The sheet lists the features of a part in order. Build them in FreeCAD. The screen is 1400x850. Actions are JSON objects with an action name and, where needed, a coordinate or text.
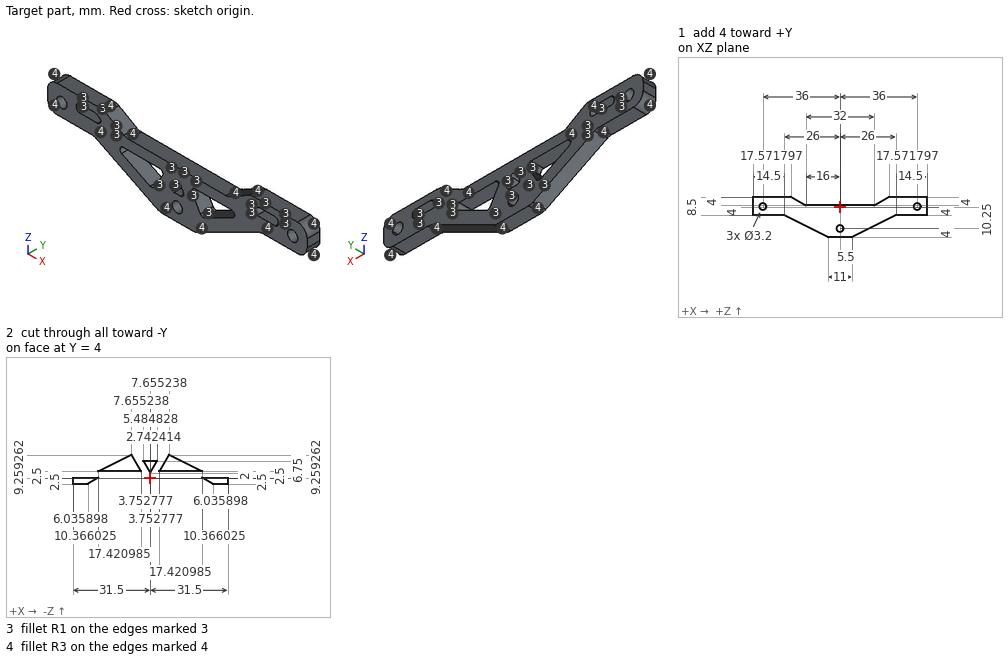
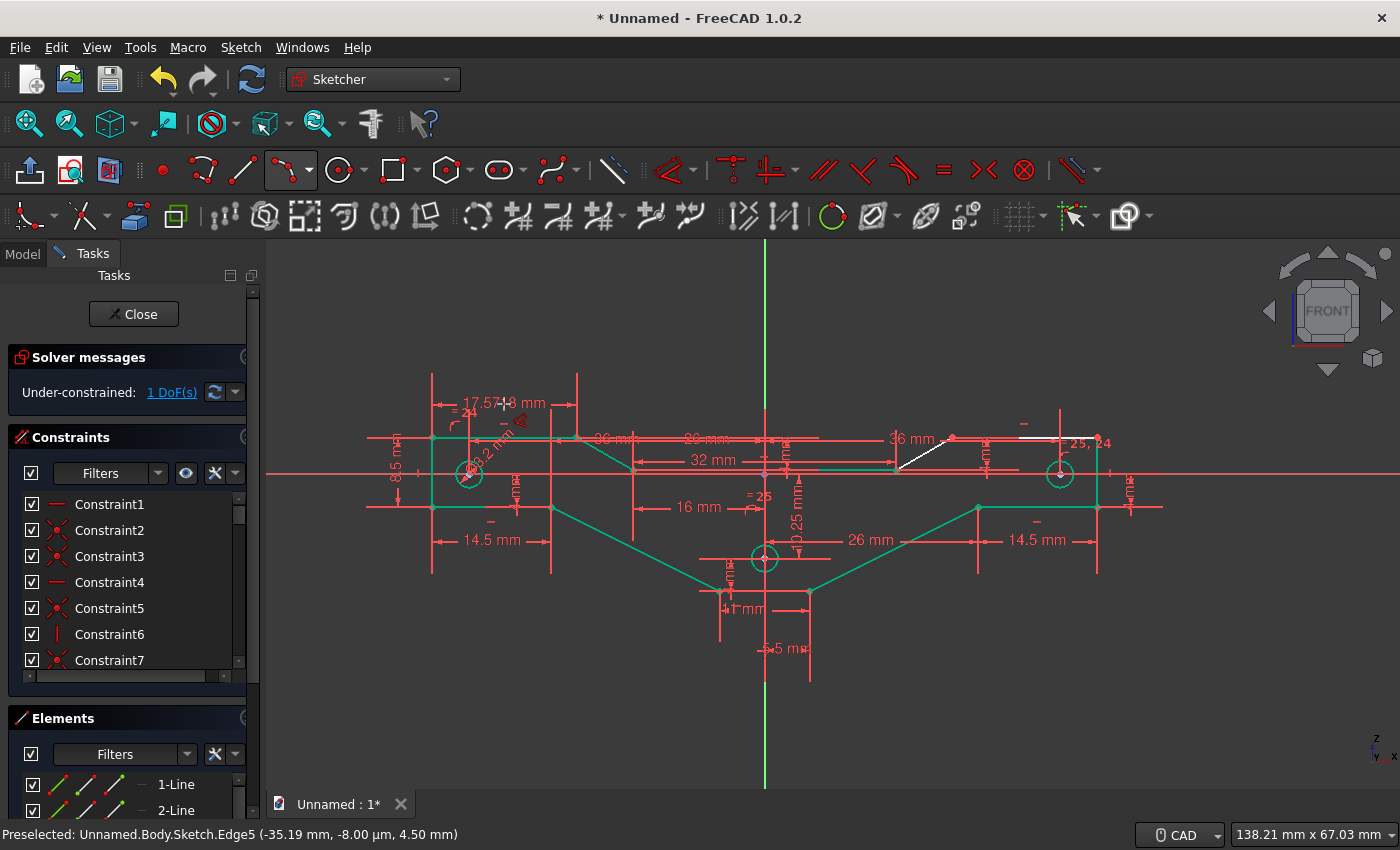
{"action": "left_click", "coordinate": [996, 438]}
{"action": "left_click", "coordinate": [1025, 404]}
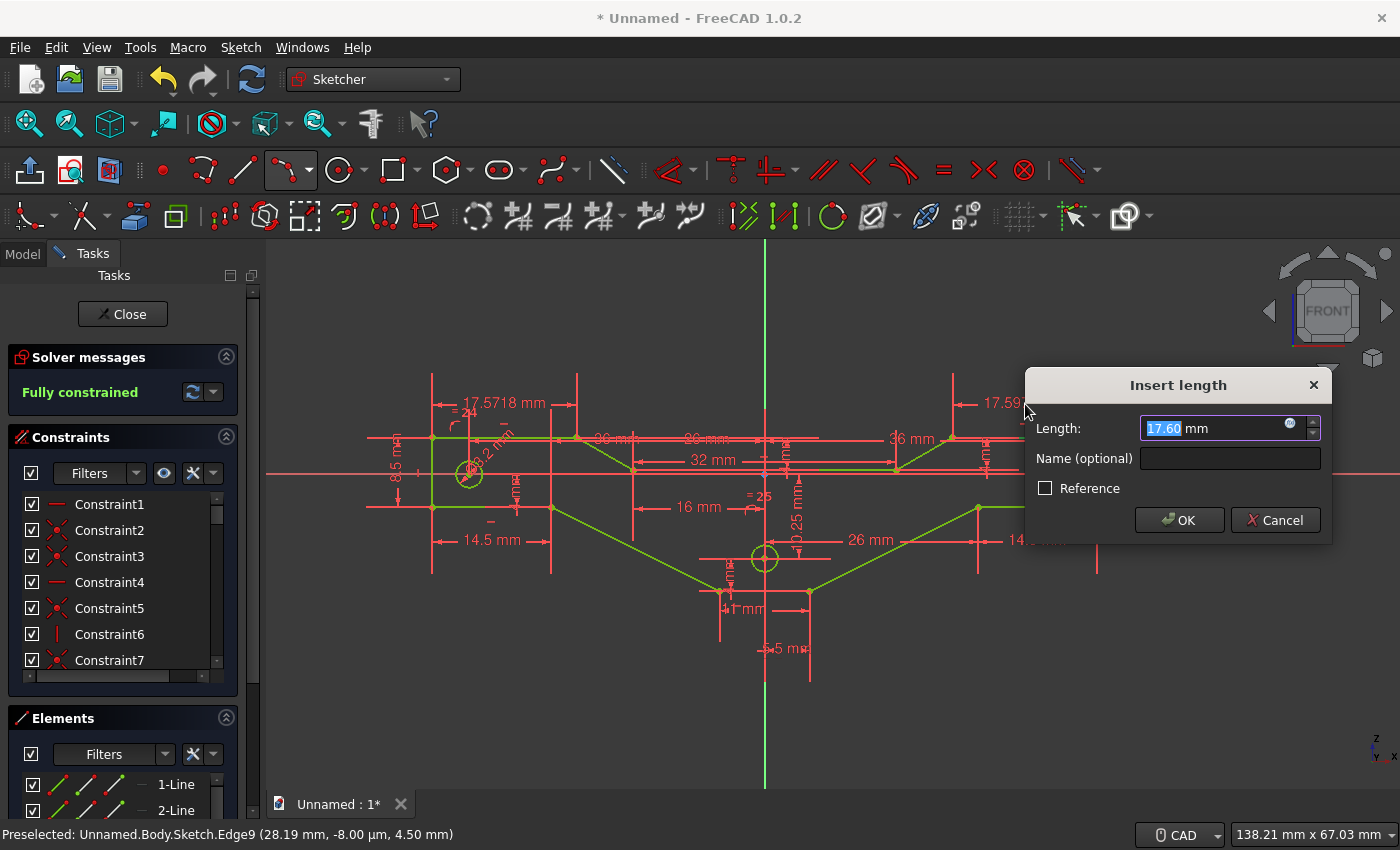
{"action": "type", "text": "17.571797"}
{"action": "key", "text": "Return"}
{"action": "key", "text": "Escape"}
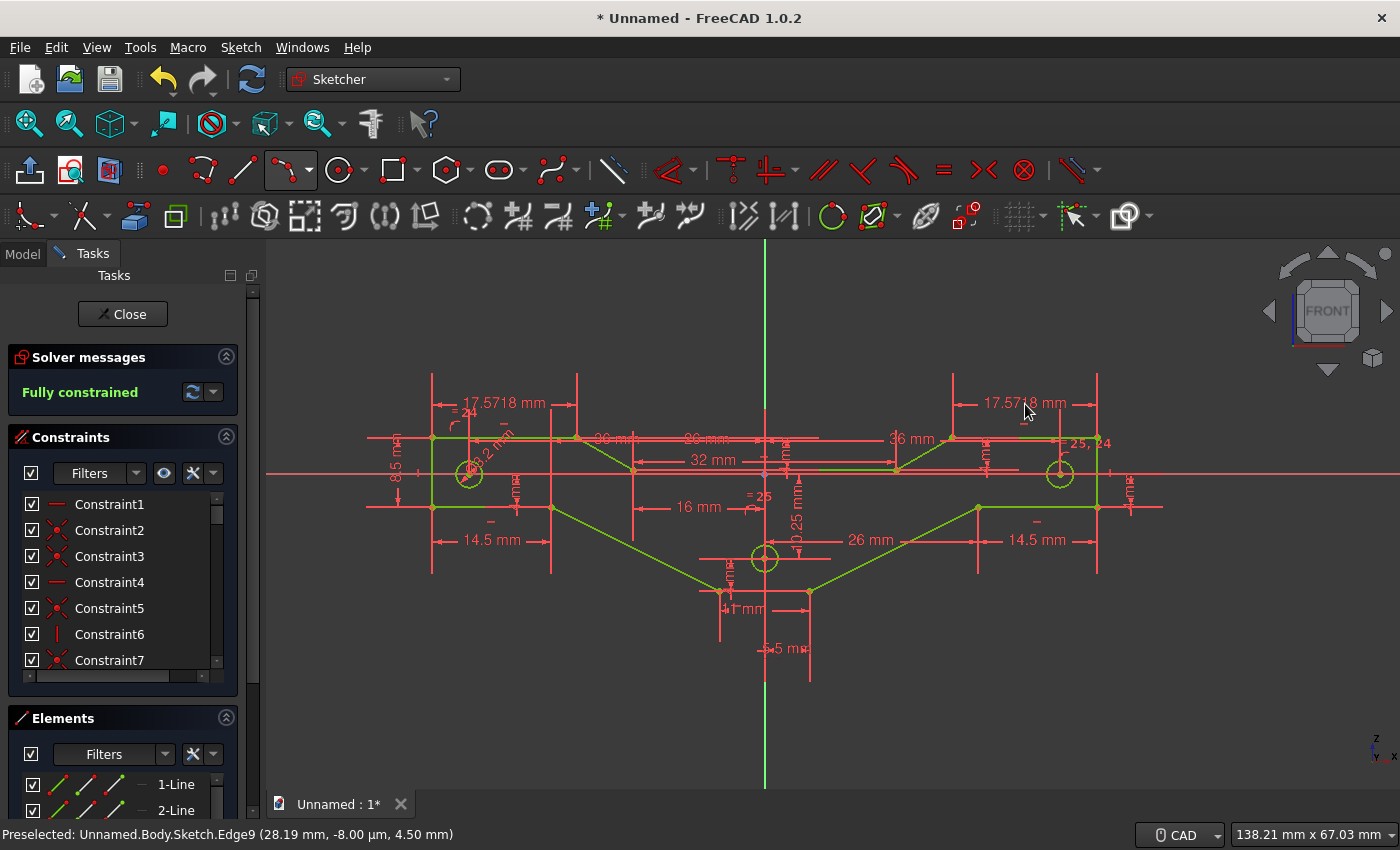
{"action": "left_click", "coordinate": [123, 314]}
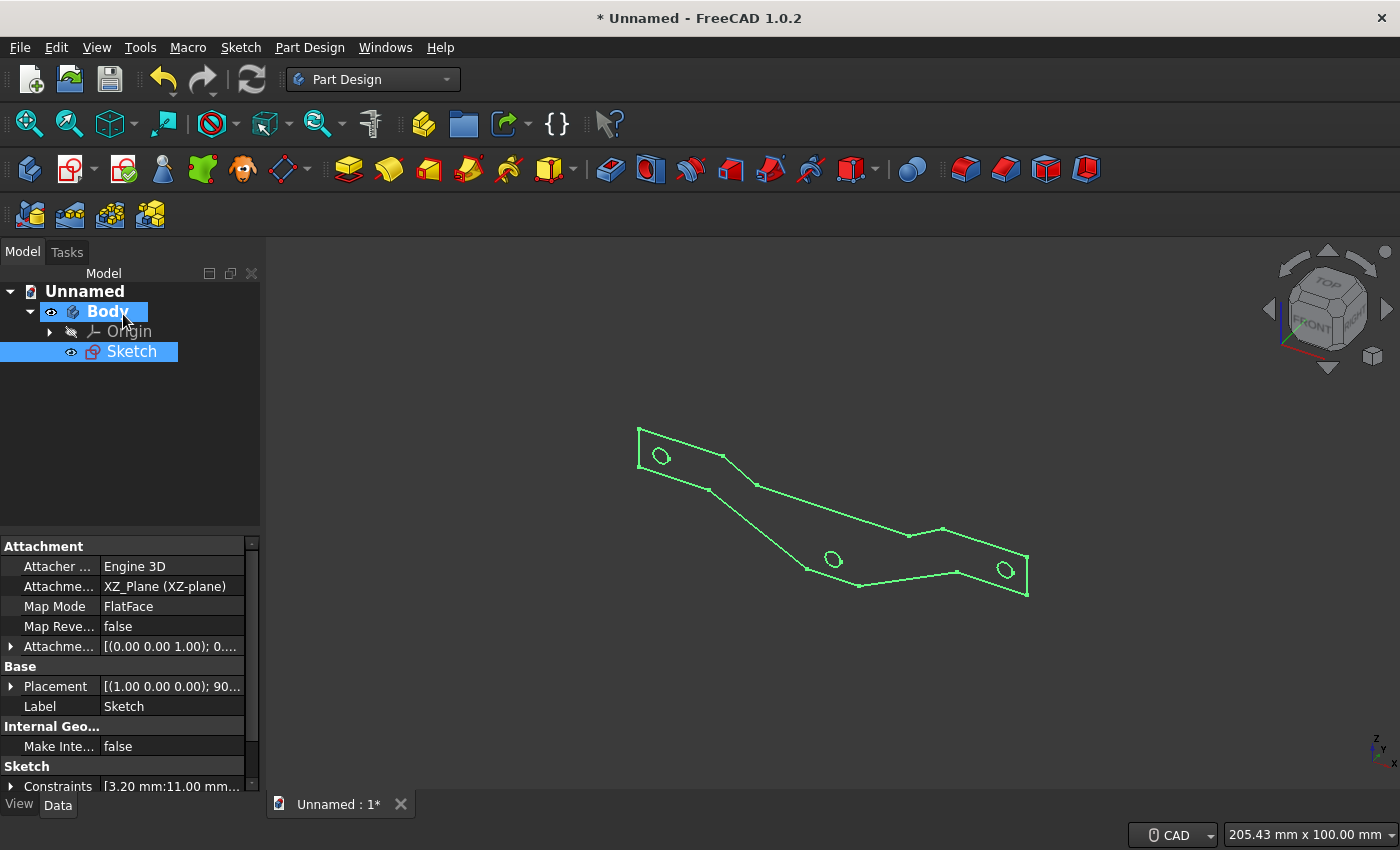
{"action": "left_click", "coordinate": [350, 170]}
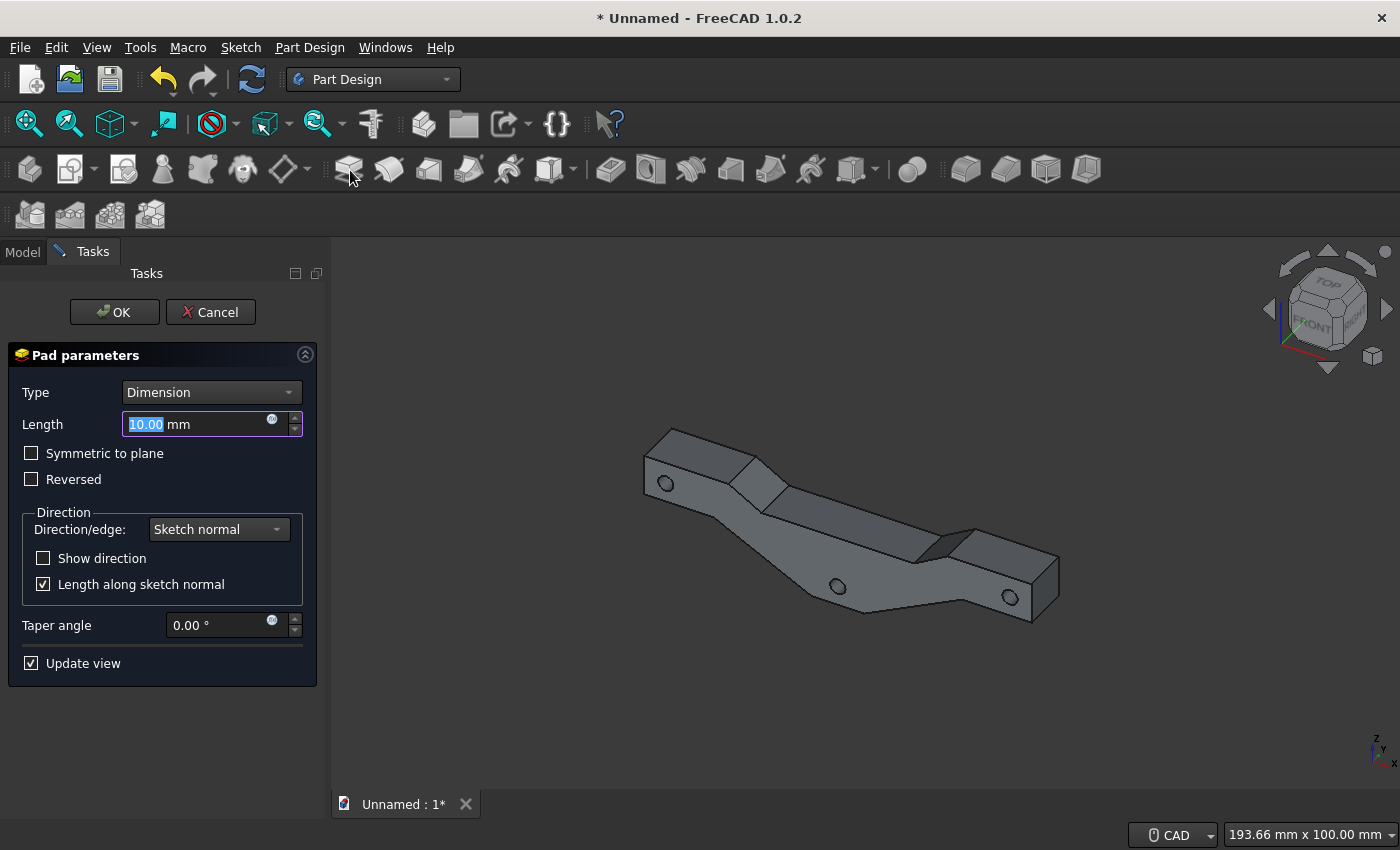
{"action": "type", "text": "4"}
{"action": "key", "text": "Tab"}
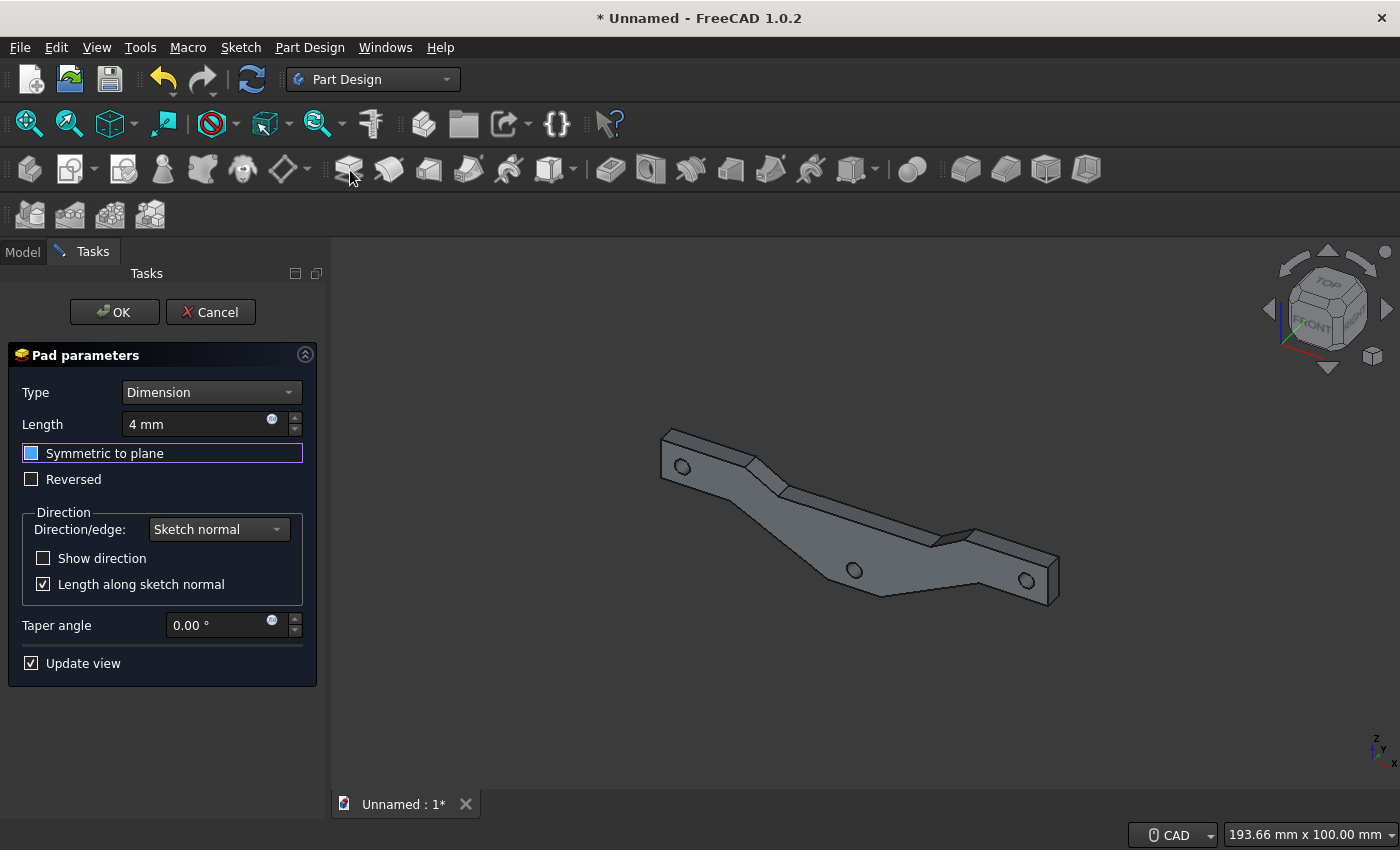
{"action": "left_click", "coordinate": [30, 479]}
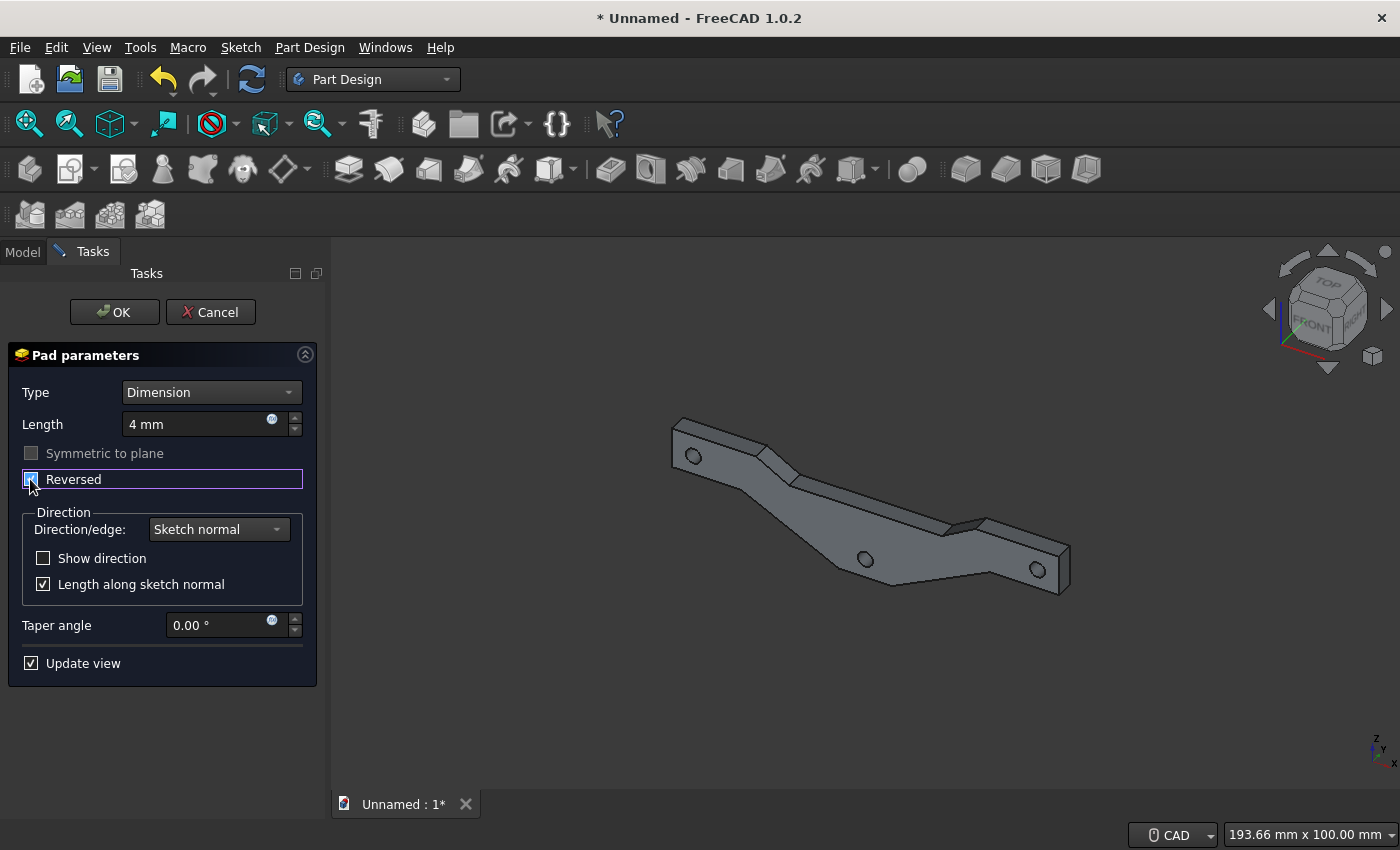
{"action": "left_click", "coordinate": [115, 312]}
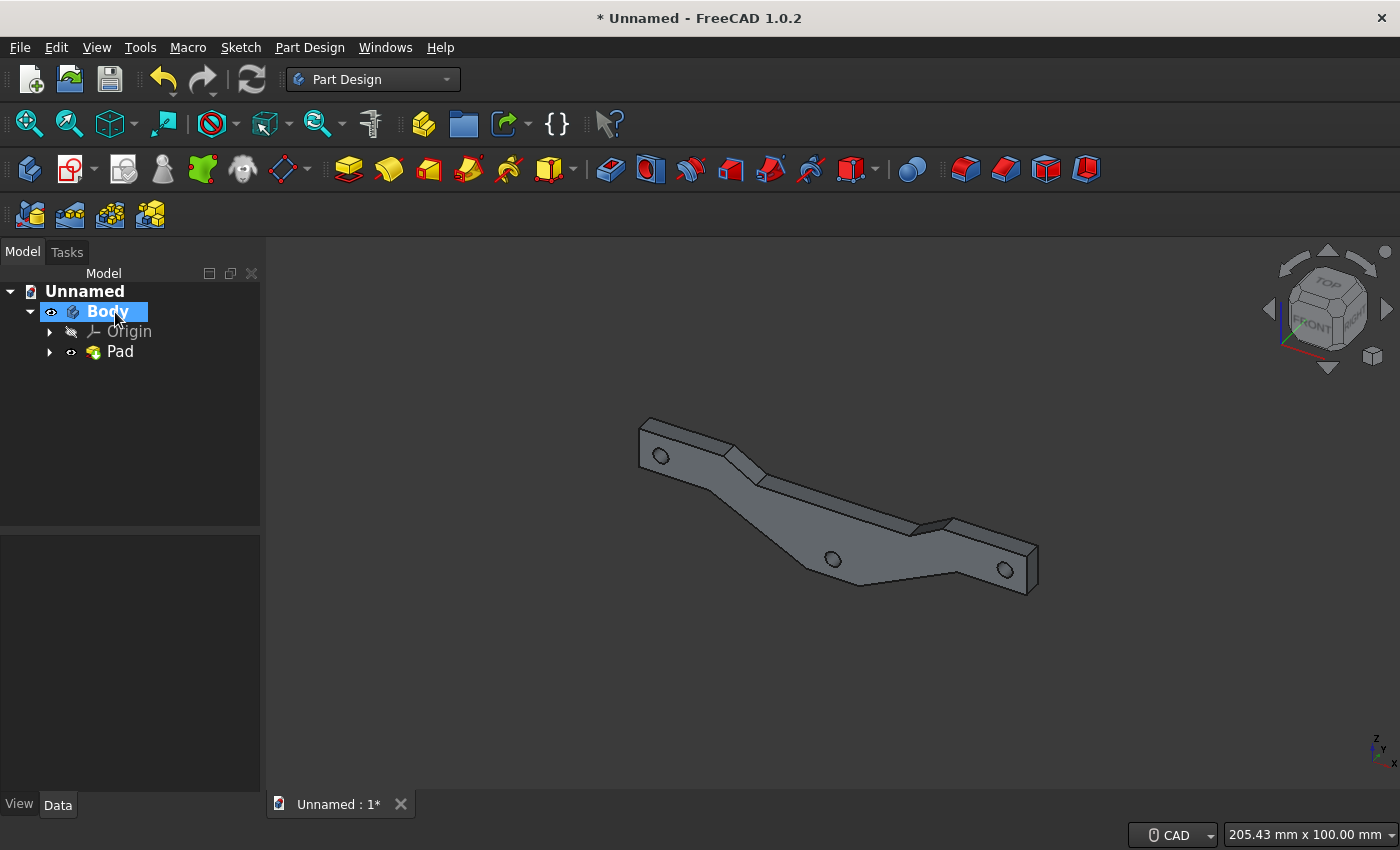
{"action": "left_click", "coordinate": [30, 124]}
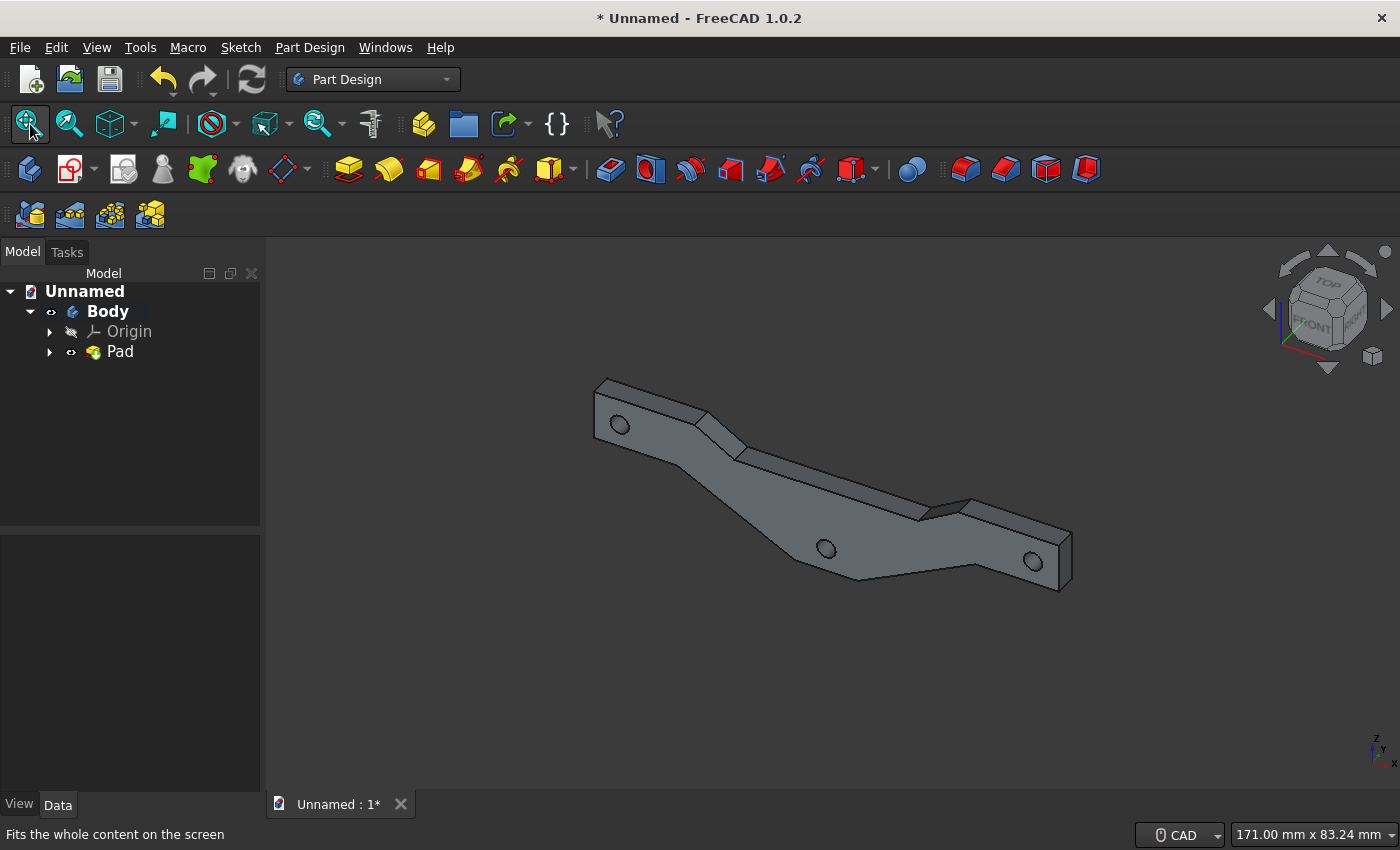
{"action": "key", "text": "4"}